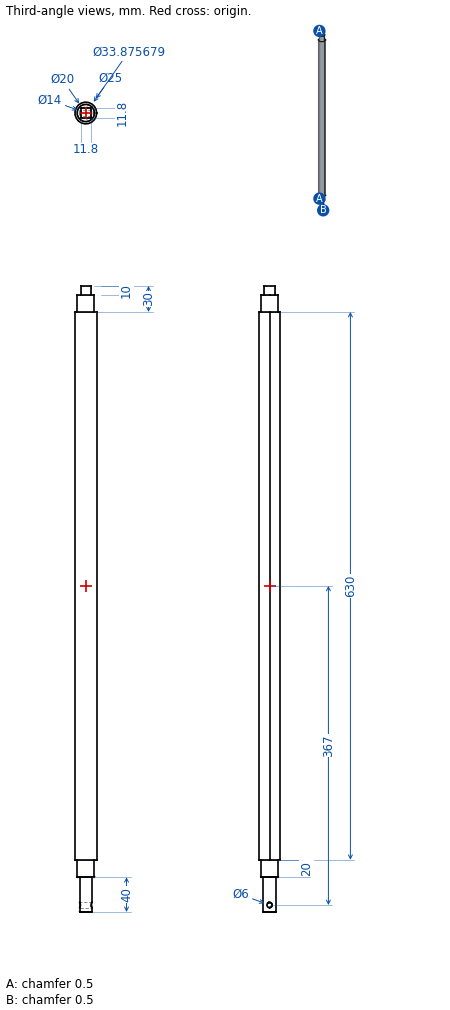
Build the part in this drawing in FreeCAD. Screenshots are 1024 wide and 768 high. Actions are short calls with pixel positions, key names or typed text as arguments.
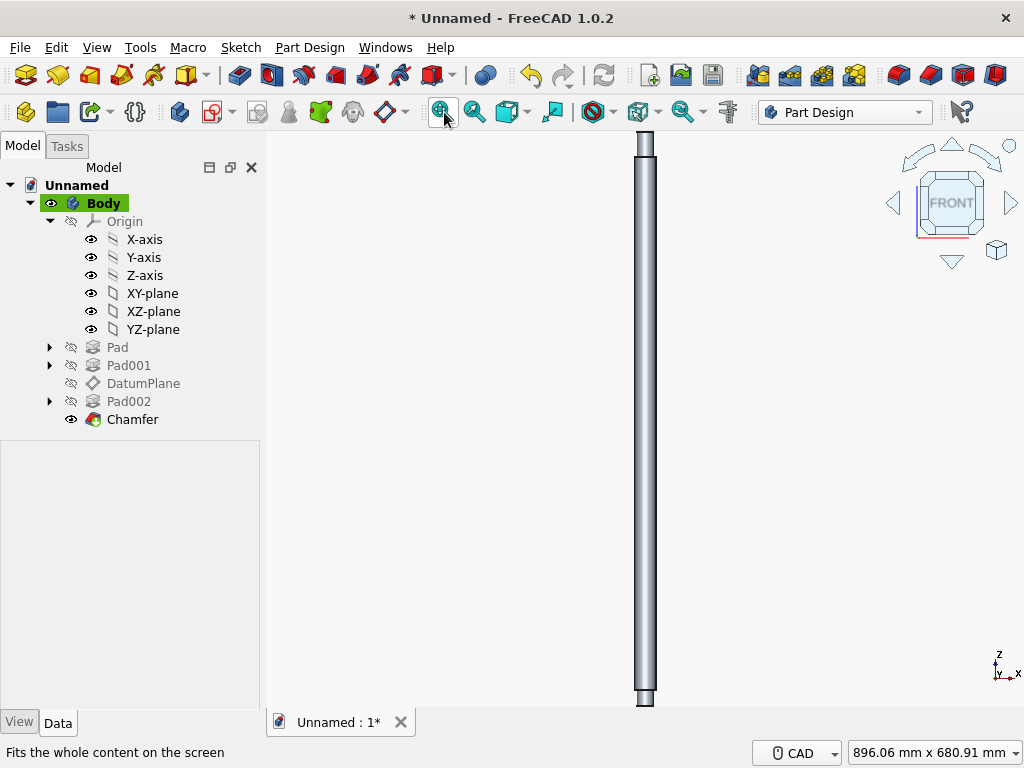
click(444, 112)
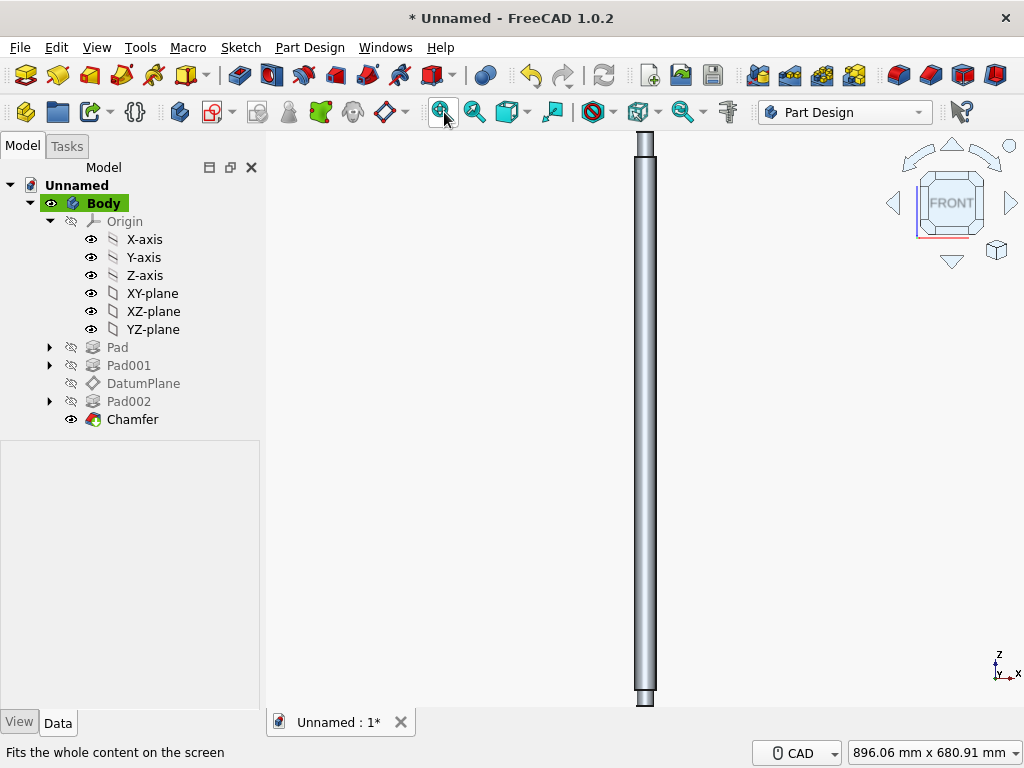
key(3)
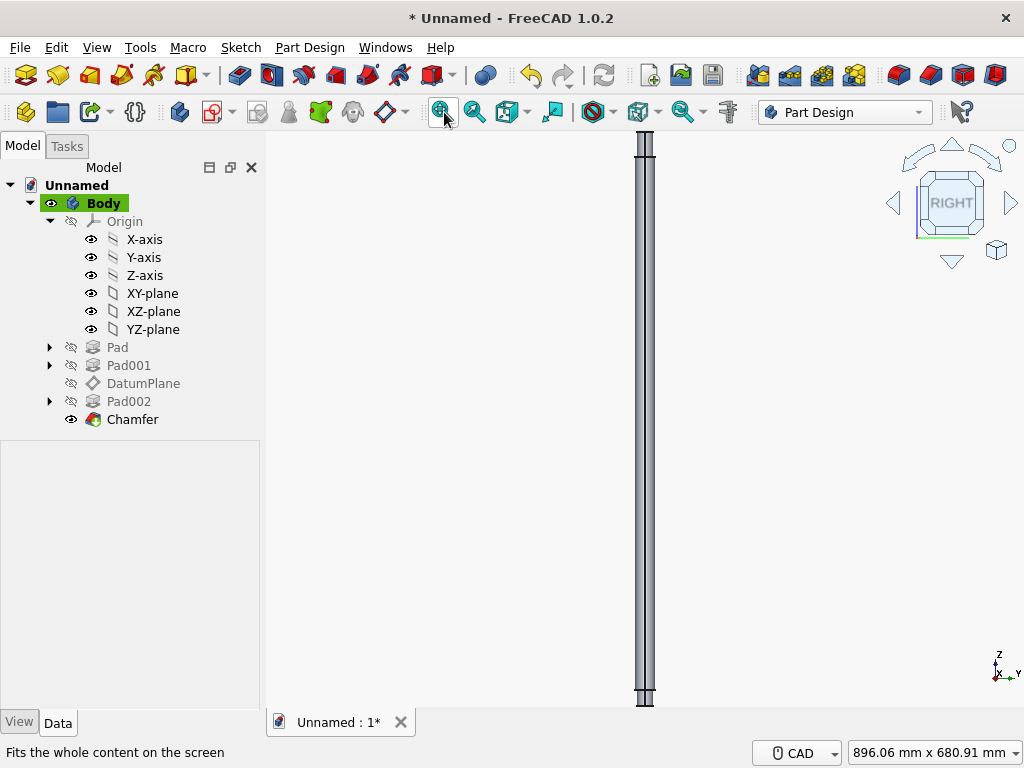
click(444, 112)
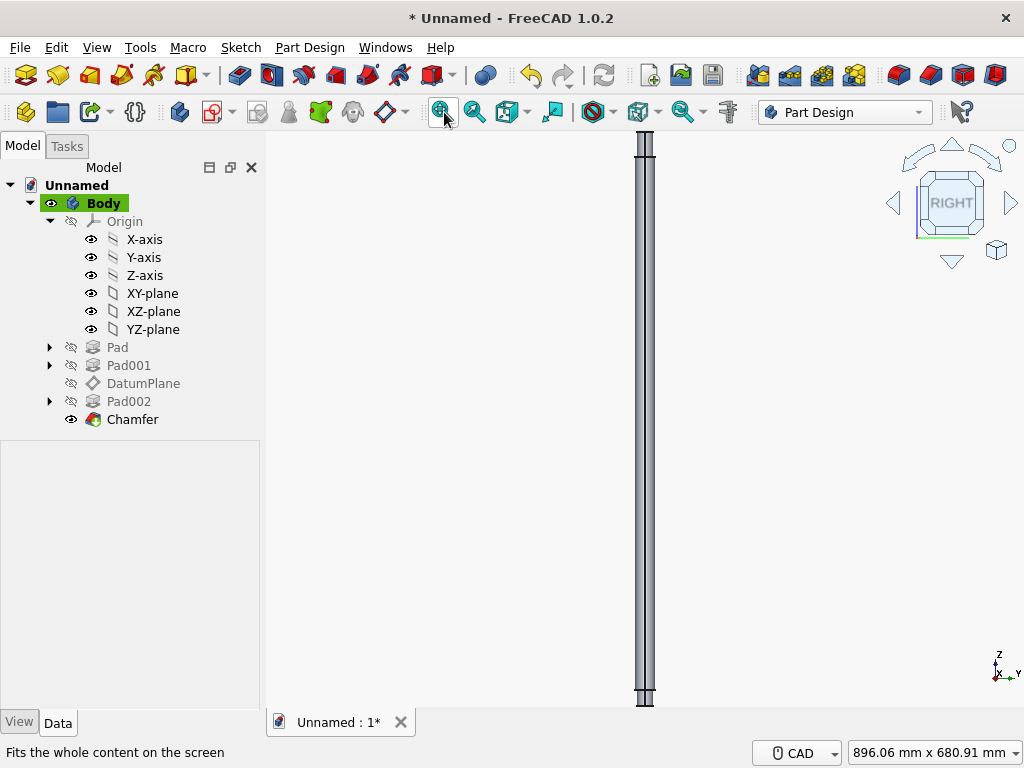
click(136, 293)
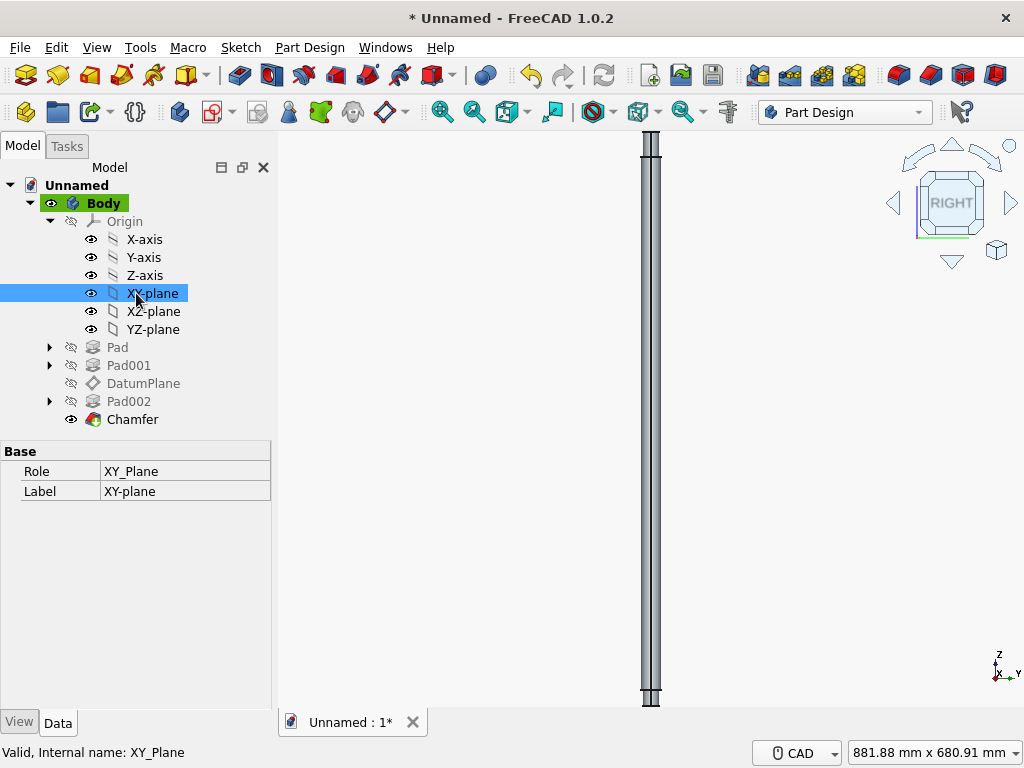
click(386, 112)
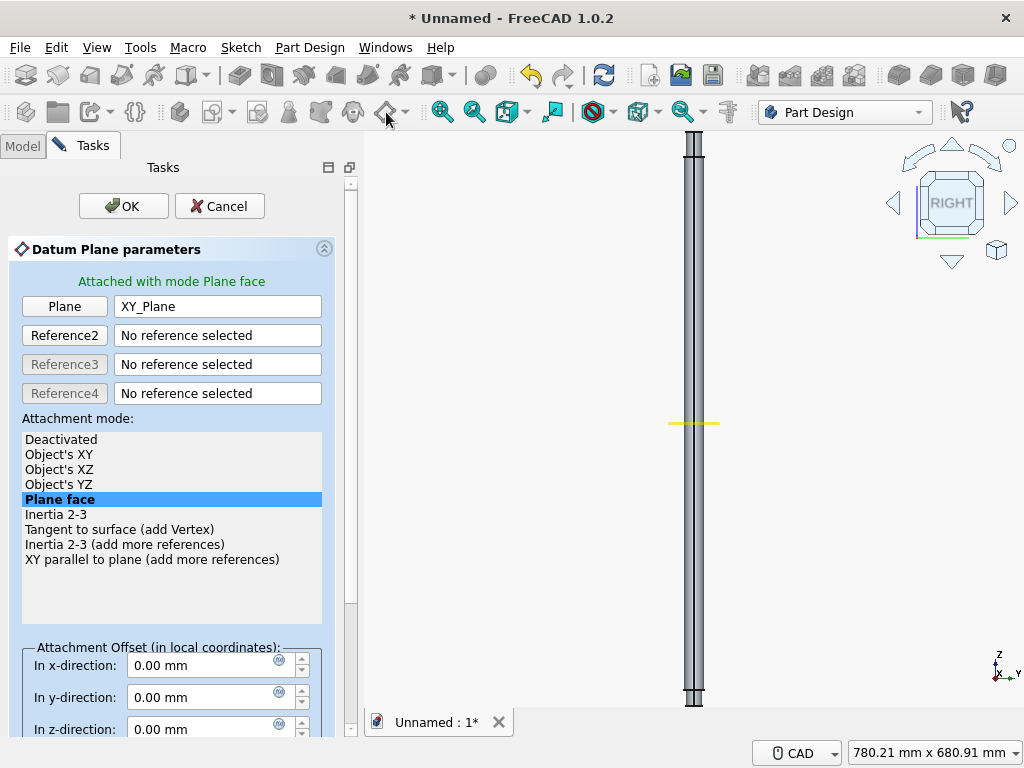
scroll(351, 456, down, 2)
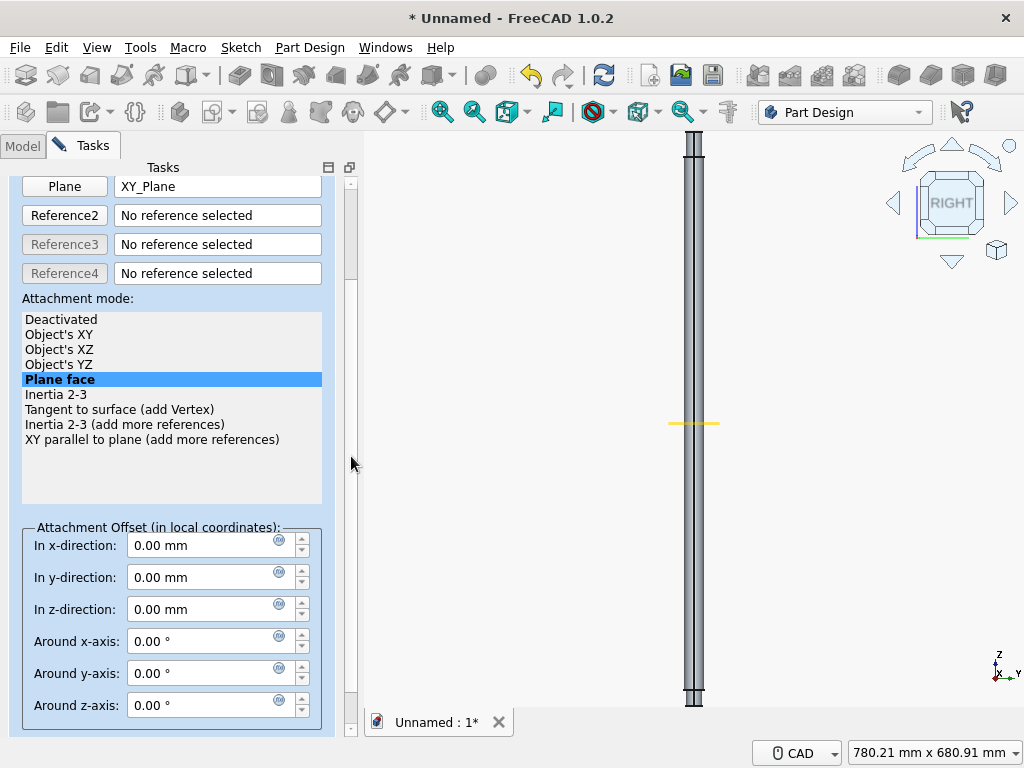
triple_click(210, 609)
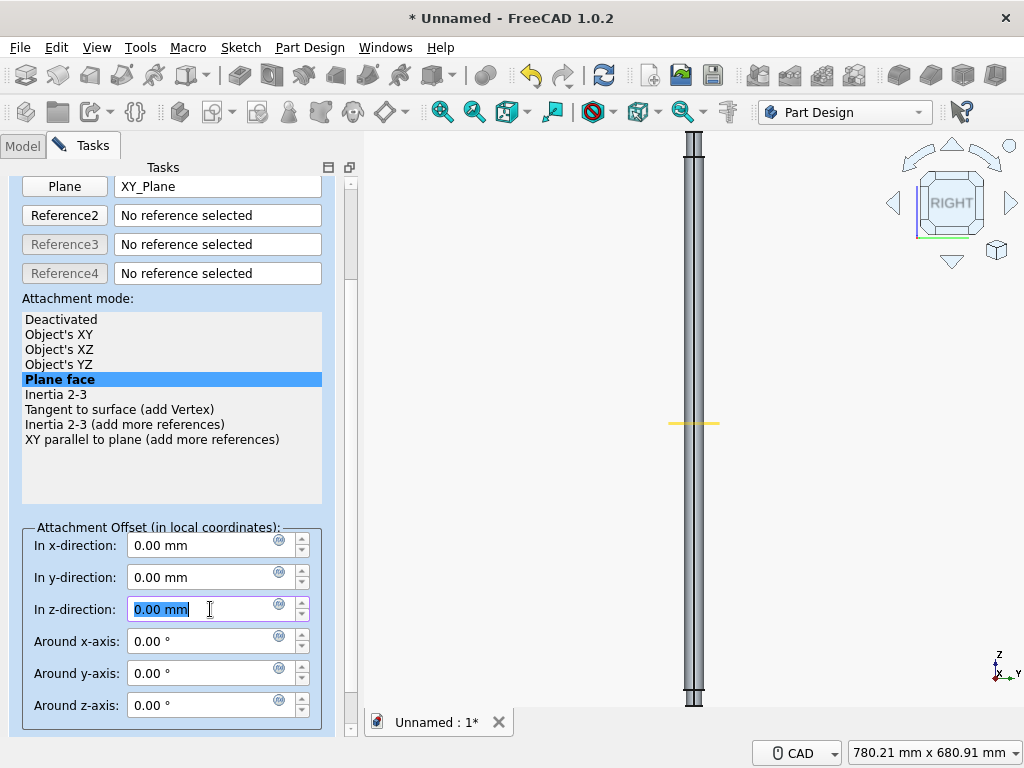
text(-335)
key(Tab)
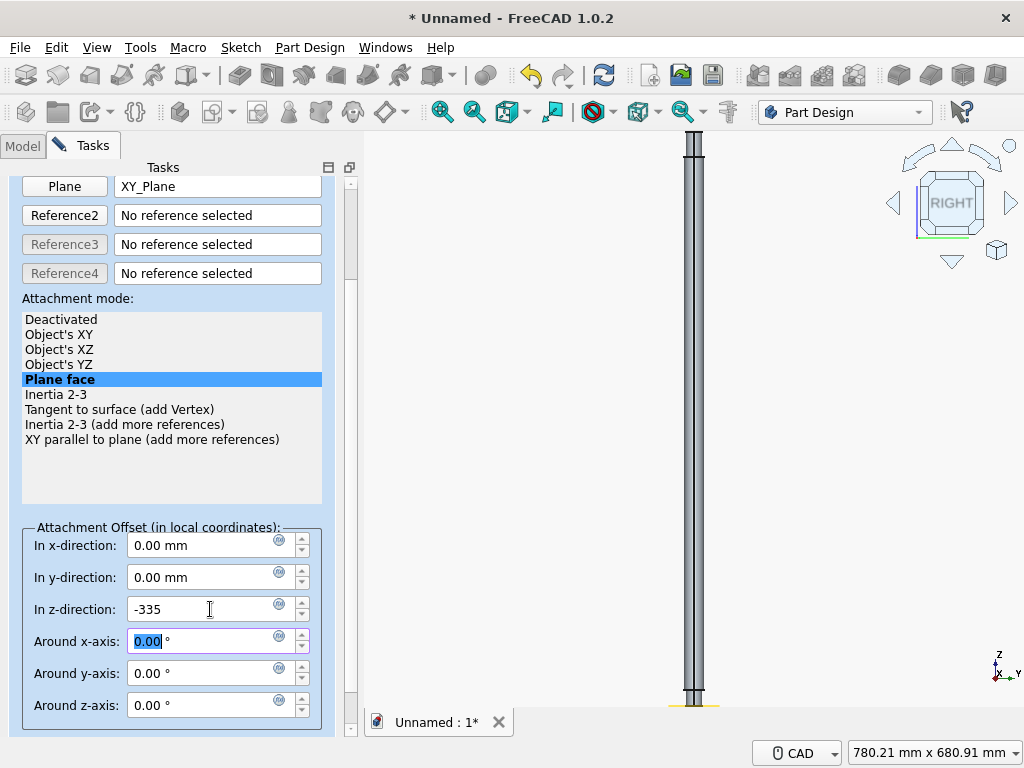
scroll(351, 456, up, 3)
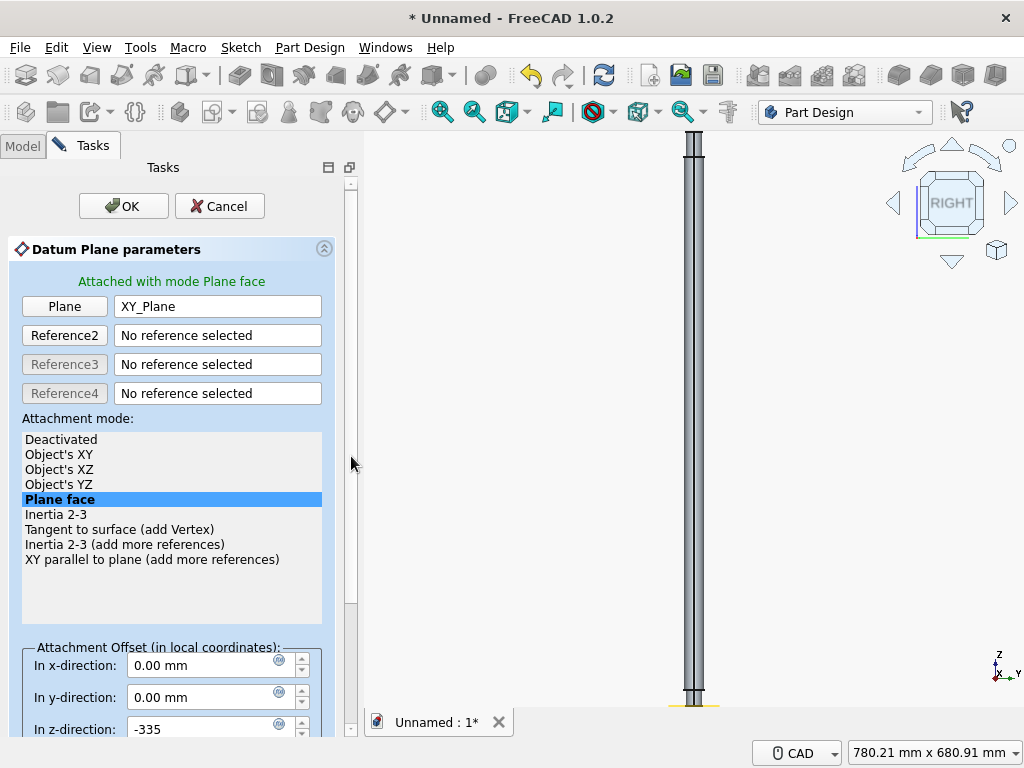
click(124, 206)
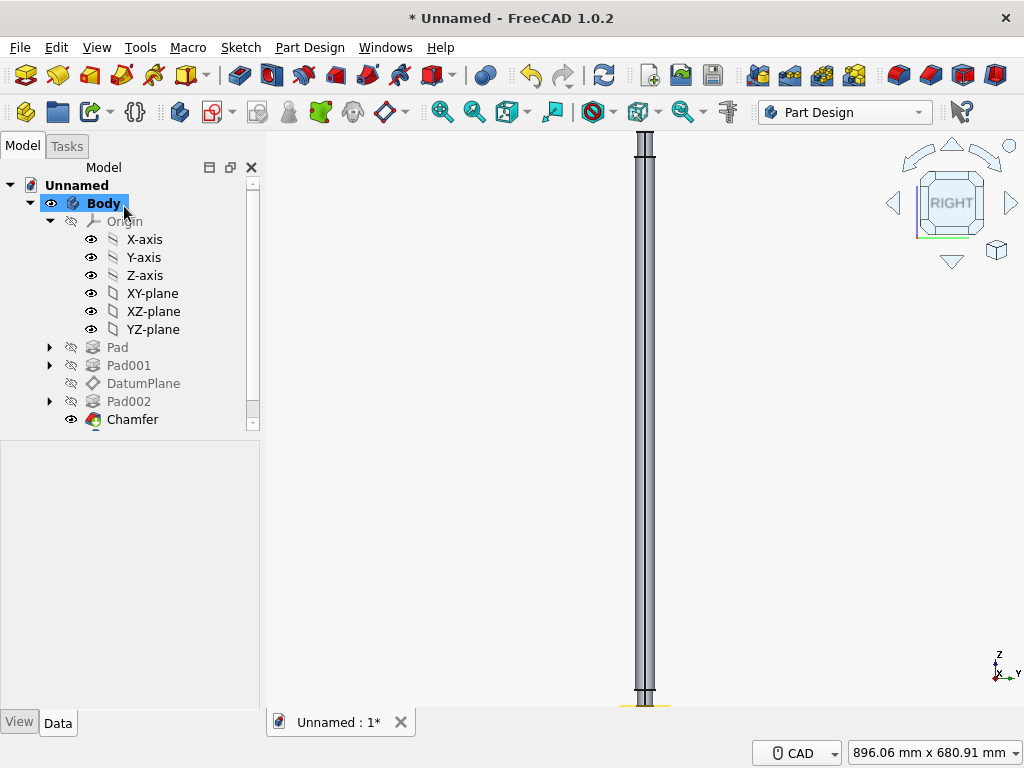
scroll(100, 307, down, 3)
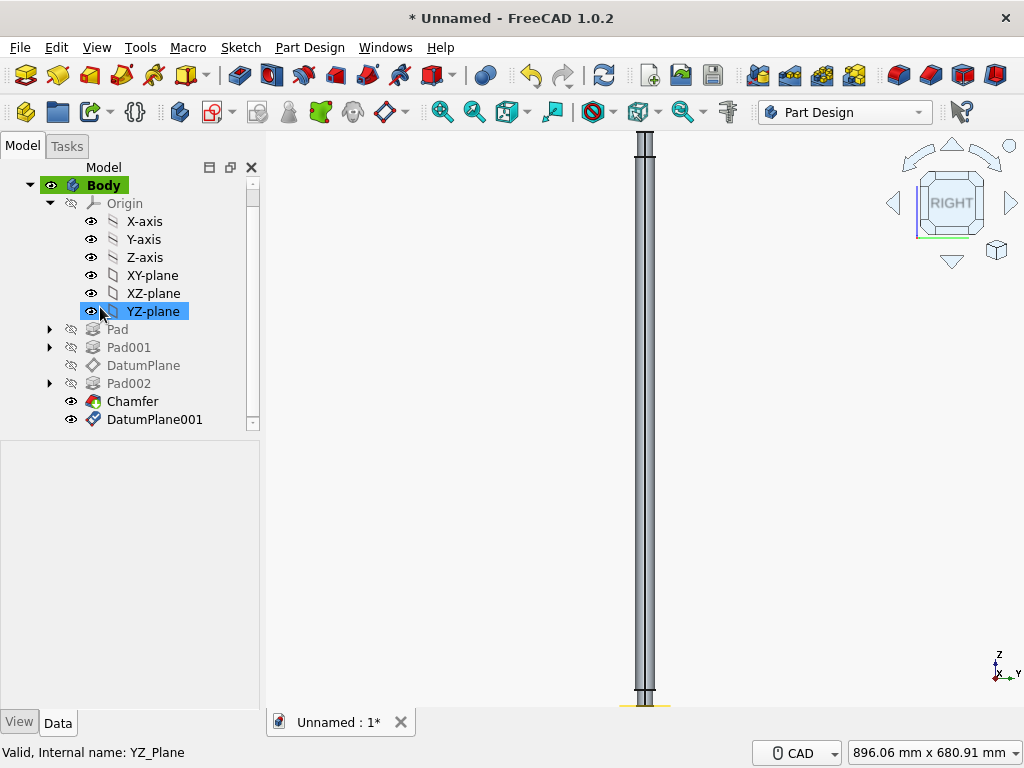
click(116, 419)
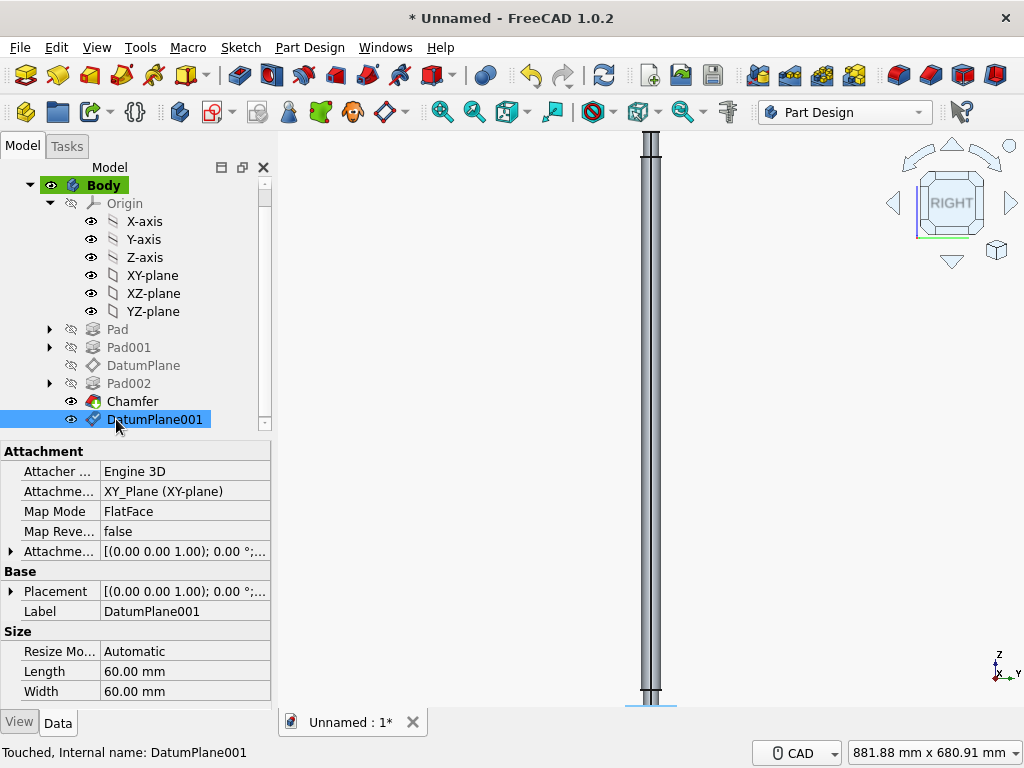
click(212, 112)